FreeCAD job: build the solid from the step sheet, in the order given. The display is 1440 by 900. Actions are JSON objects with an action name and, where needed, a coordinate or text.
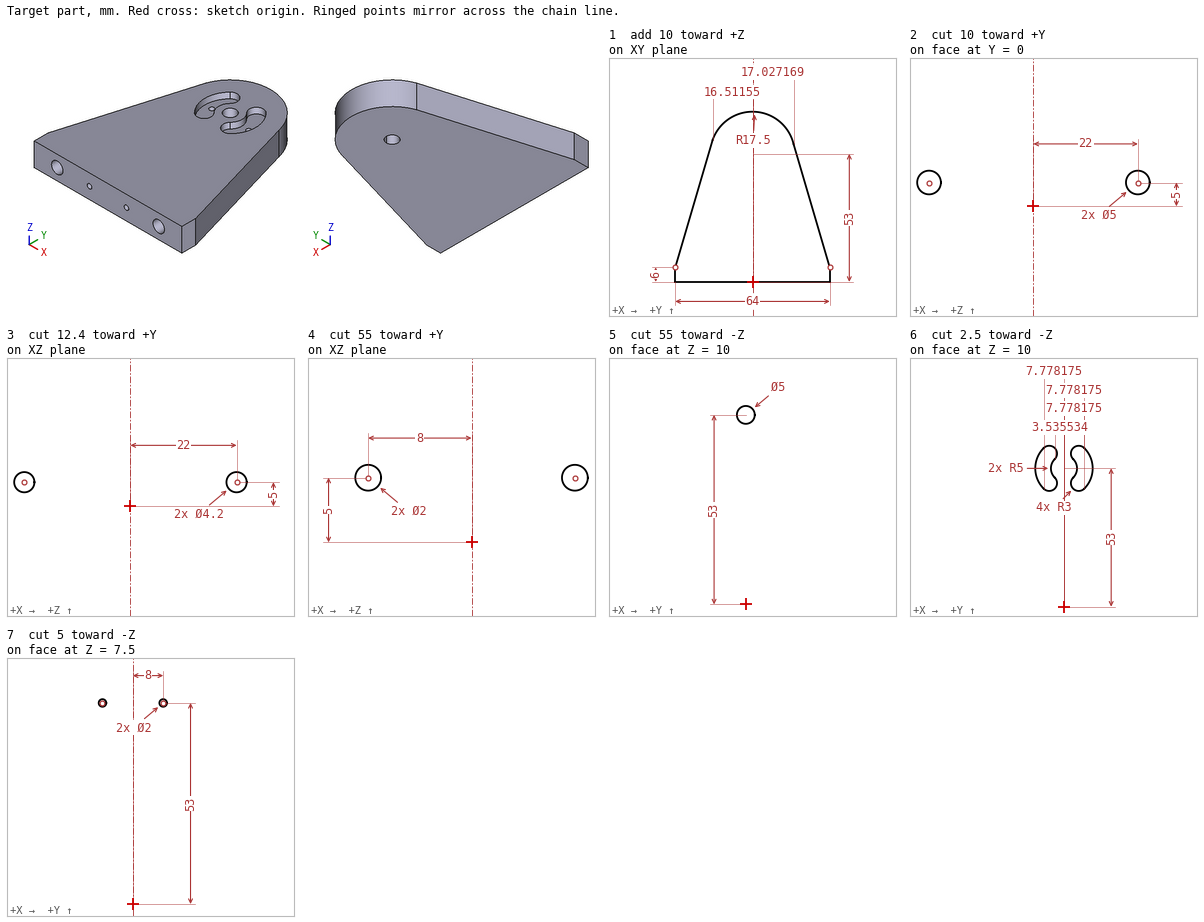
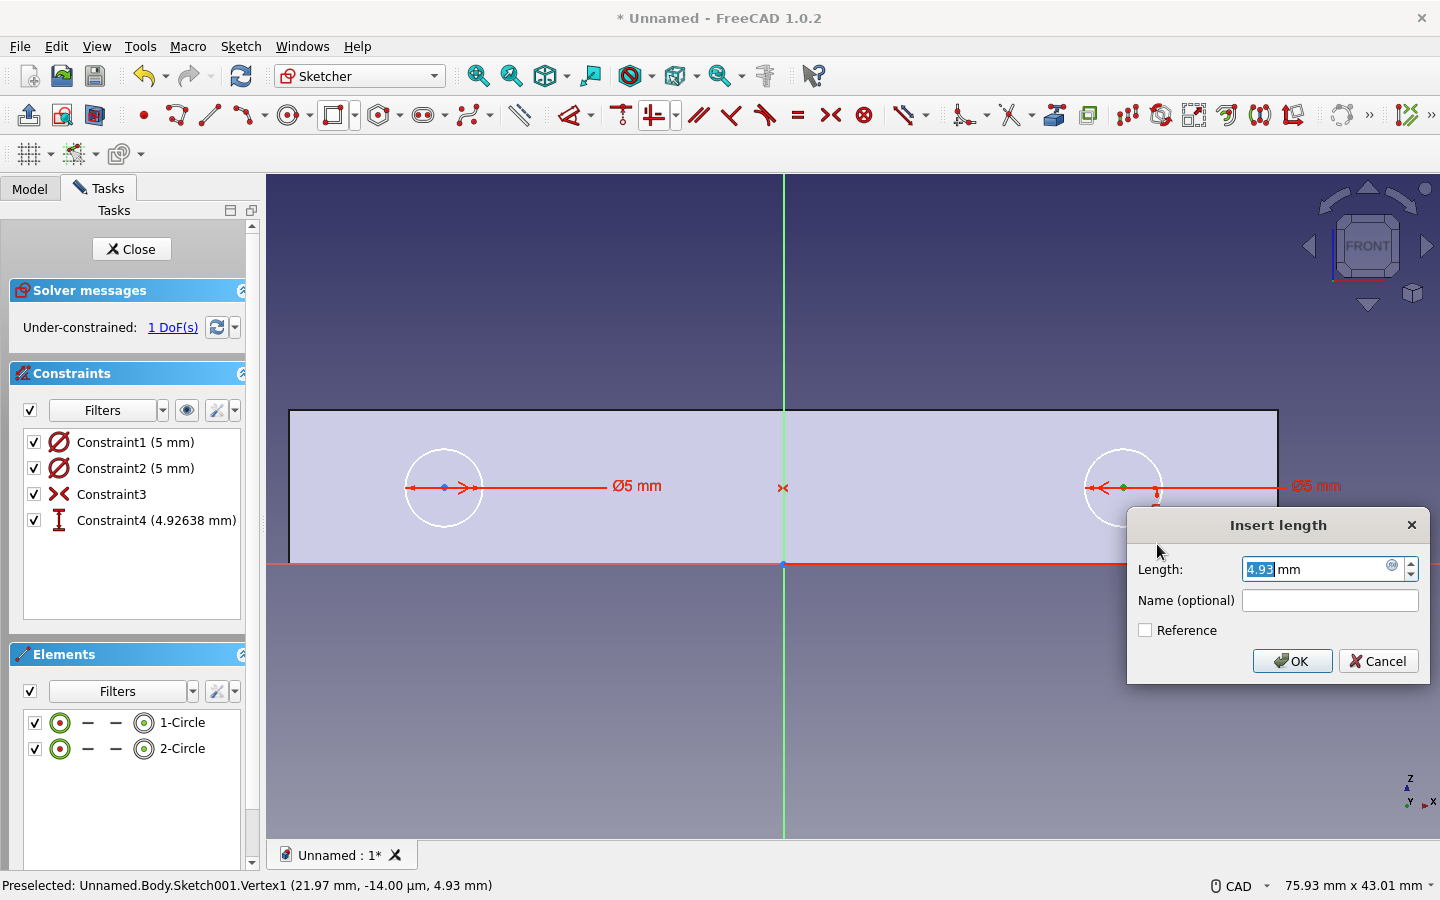
{"action": "type", "text": "5"}
{"action": "key", "text": "Return"}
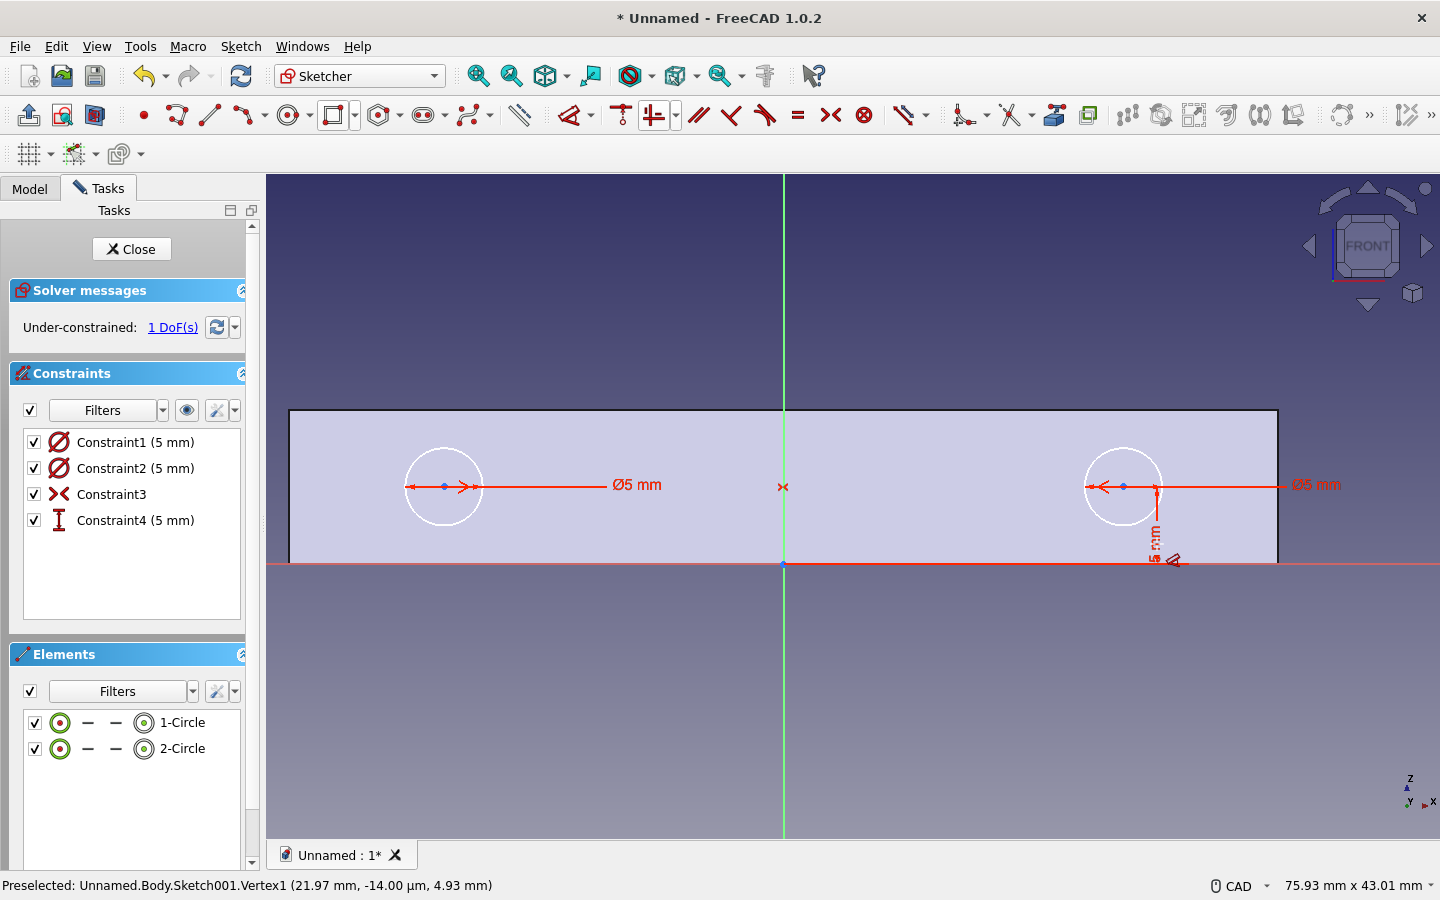
{"action": "left_click", "coordinate": [1123, 487]}
{"action": "left_click", "coordinate": [954, 598]}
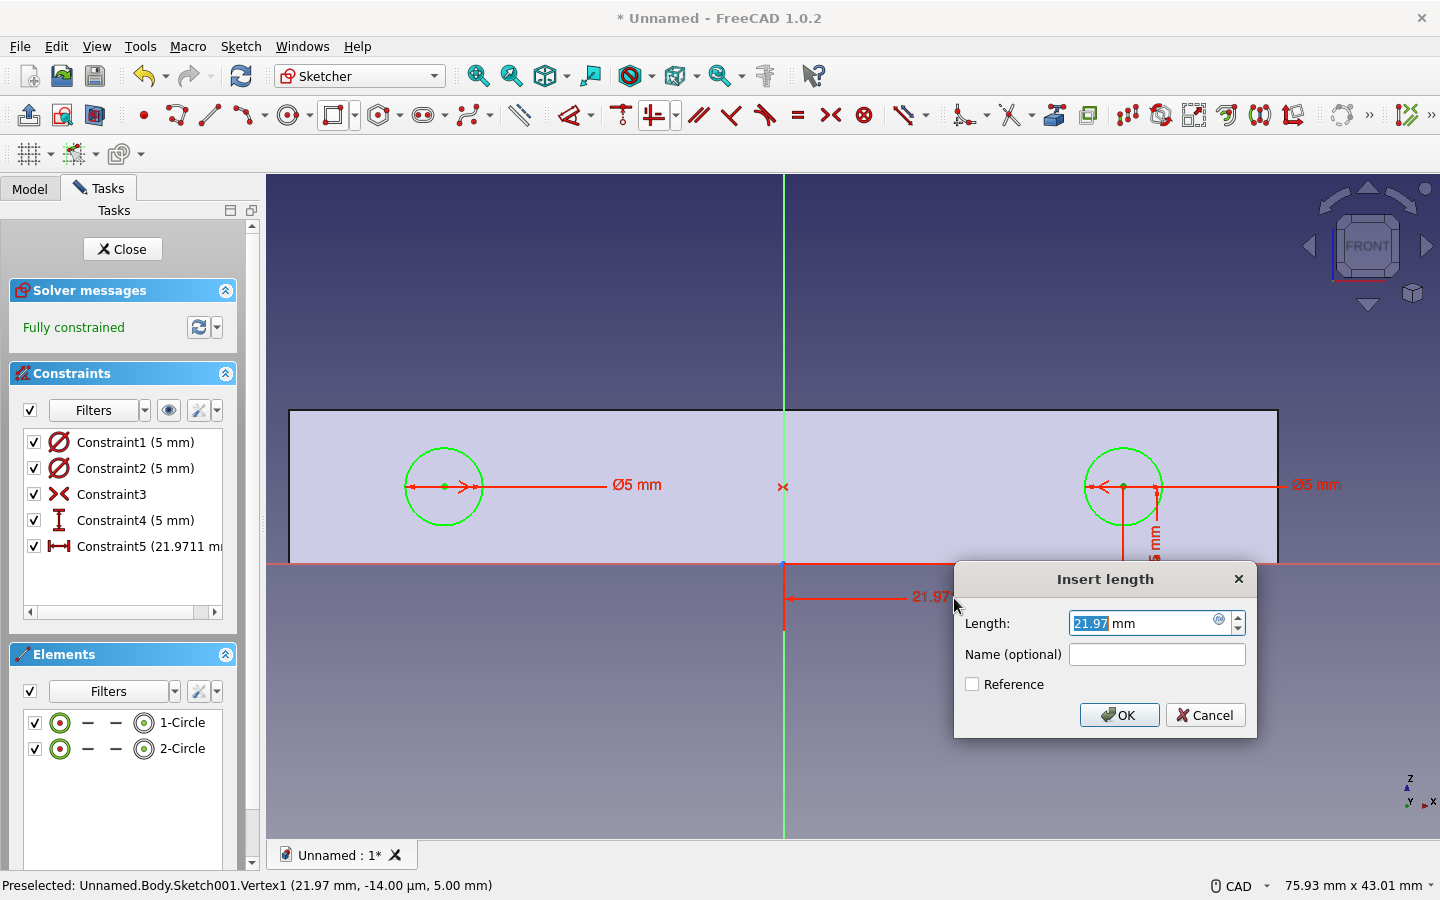
{"action": "type", "text": "22"}
{"action": "key", "text": "Return"}
{"action": "key", "text": "Escape"}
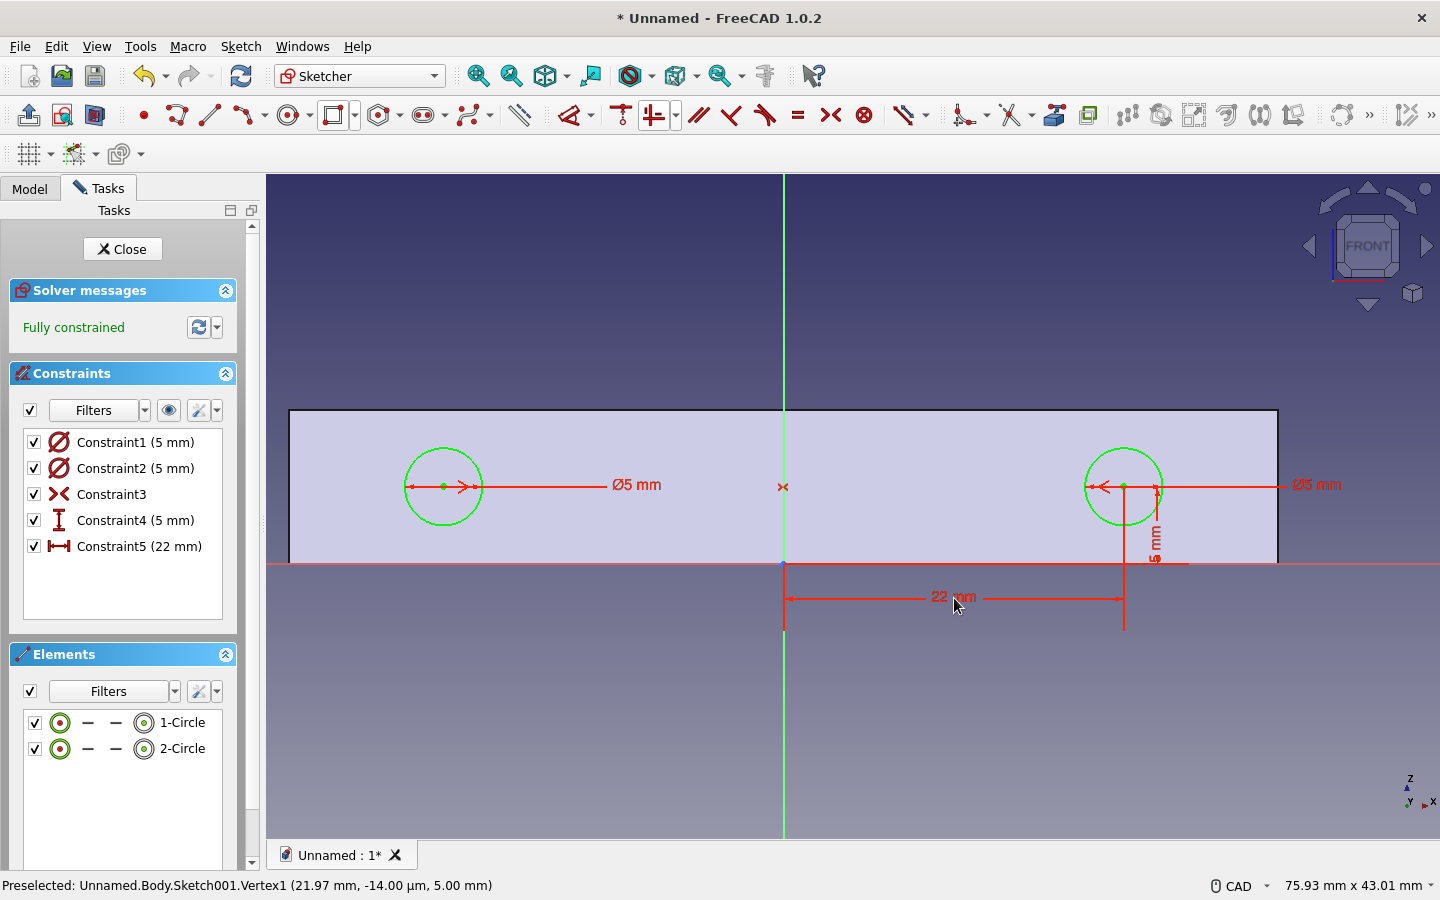
{"action": "left_click", "coordinate": [123, 249]}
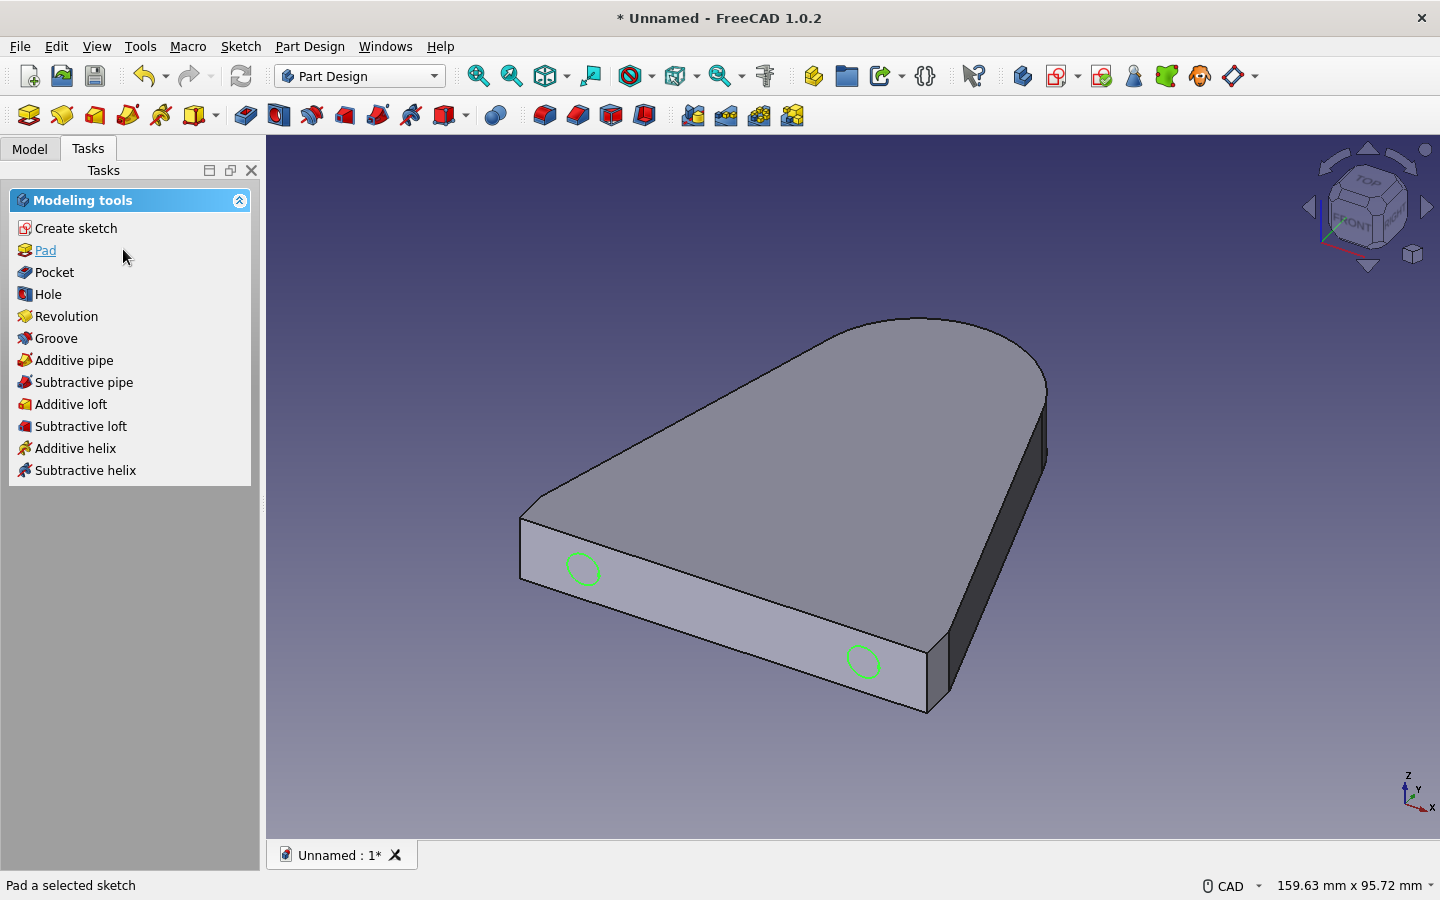
{"action": "left_click", "coordinate": [246, 116]}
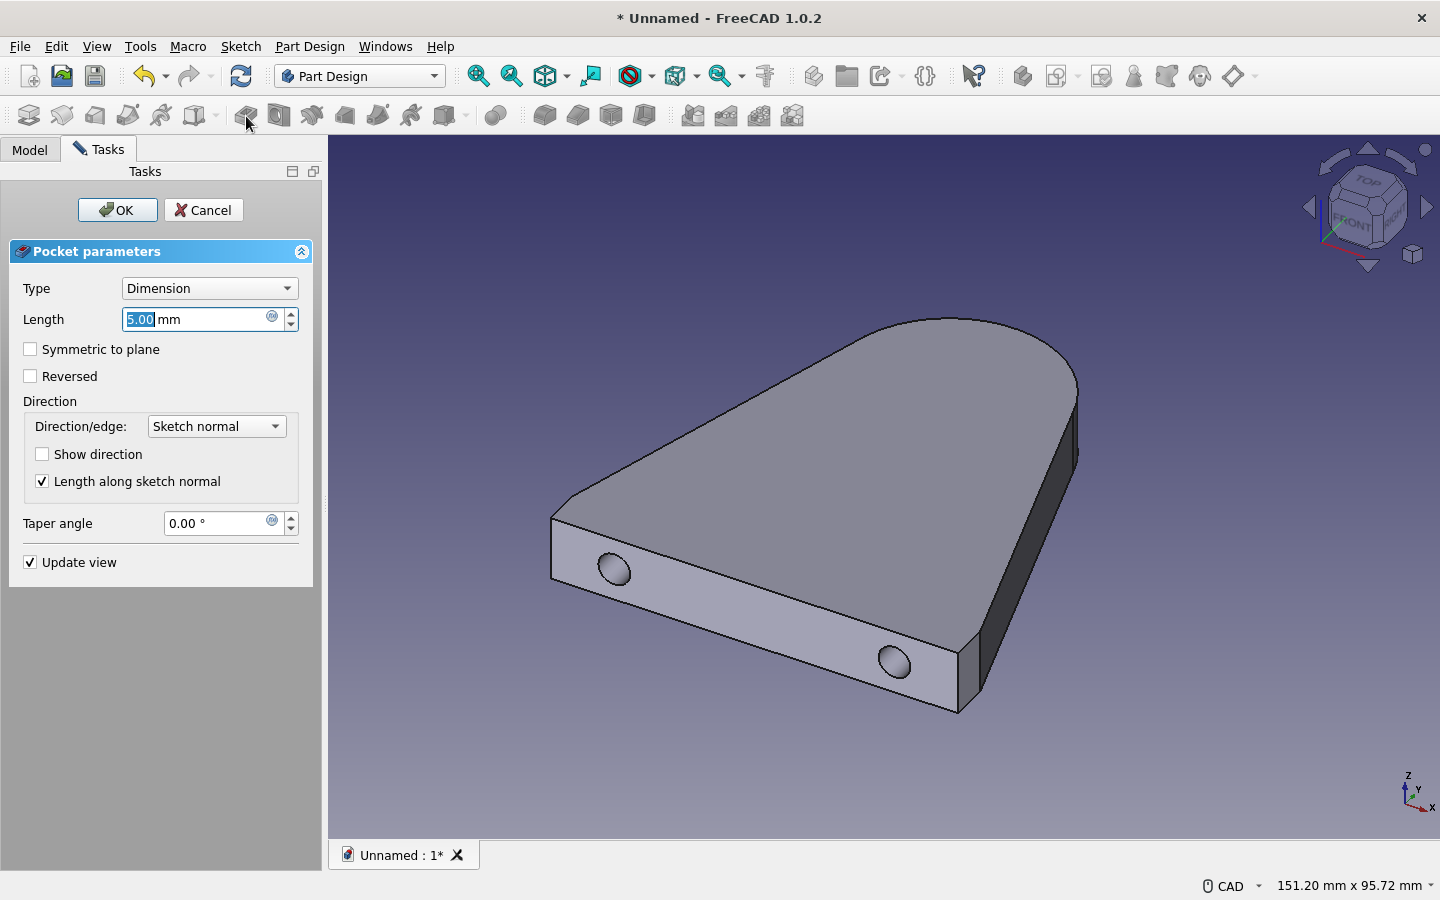
{"action": "type", "text": "10"}
{"action": "key", "text": "Tab"}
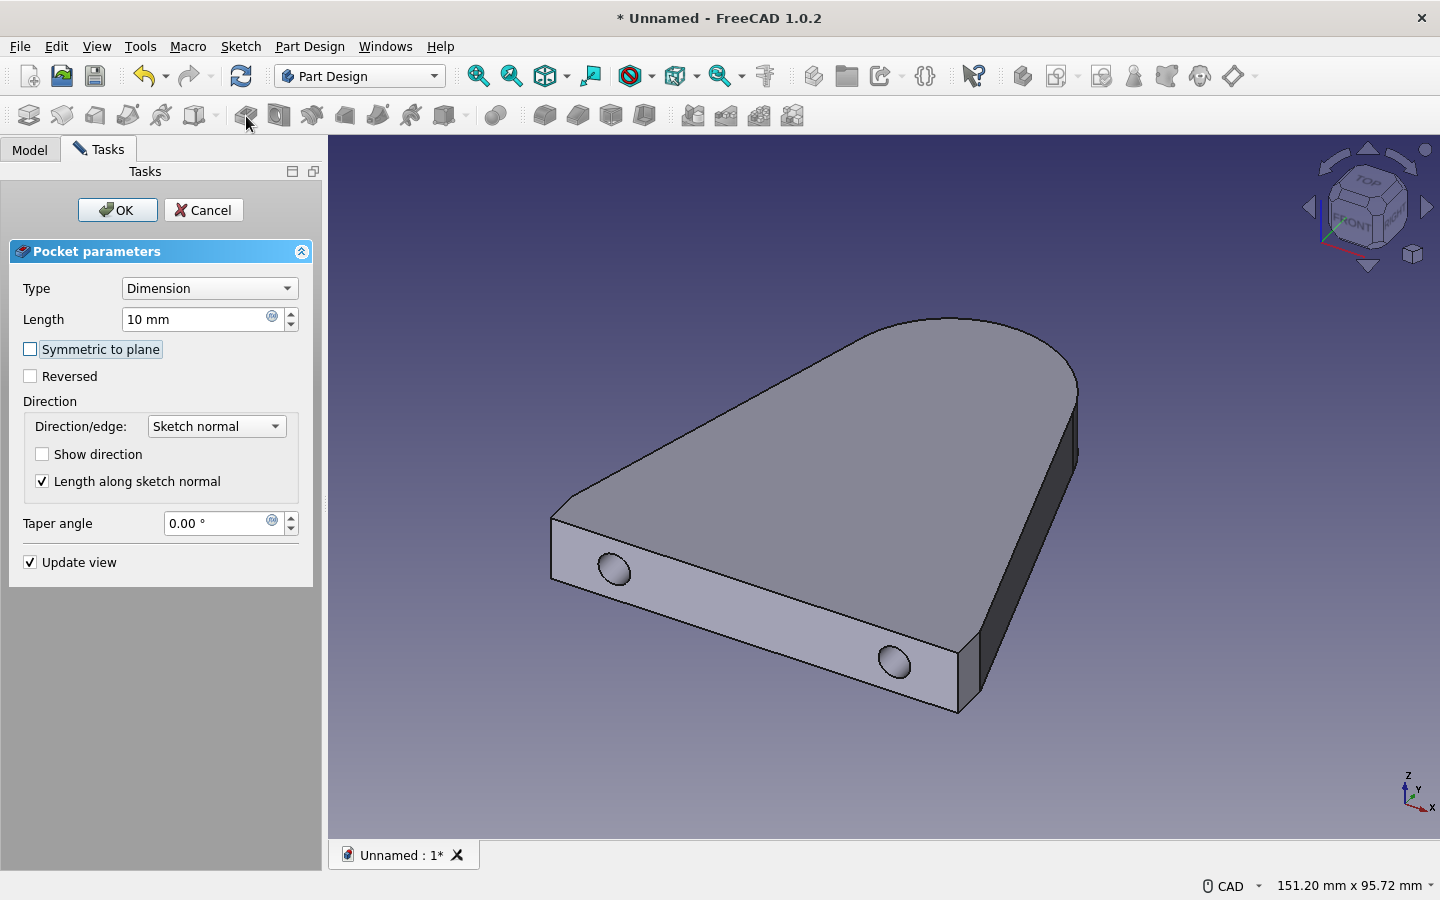
{"action": "left_click", "coordinate": [118, 210]}